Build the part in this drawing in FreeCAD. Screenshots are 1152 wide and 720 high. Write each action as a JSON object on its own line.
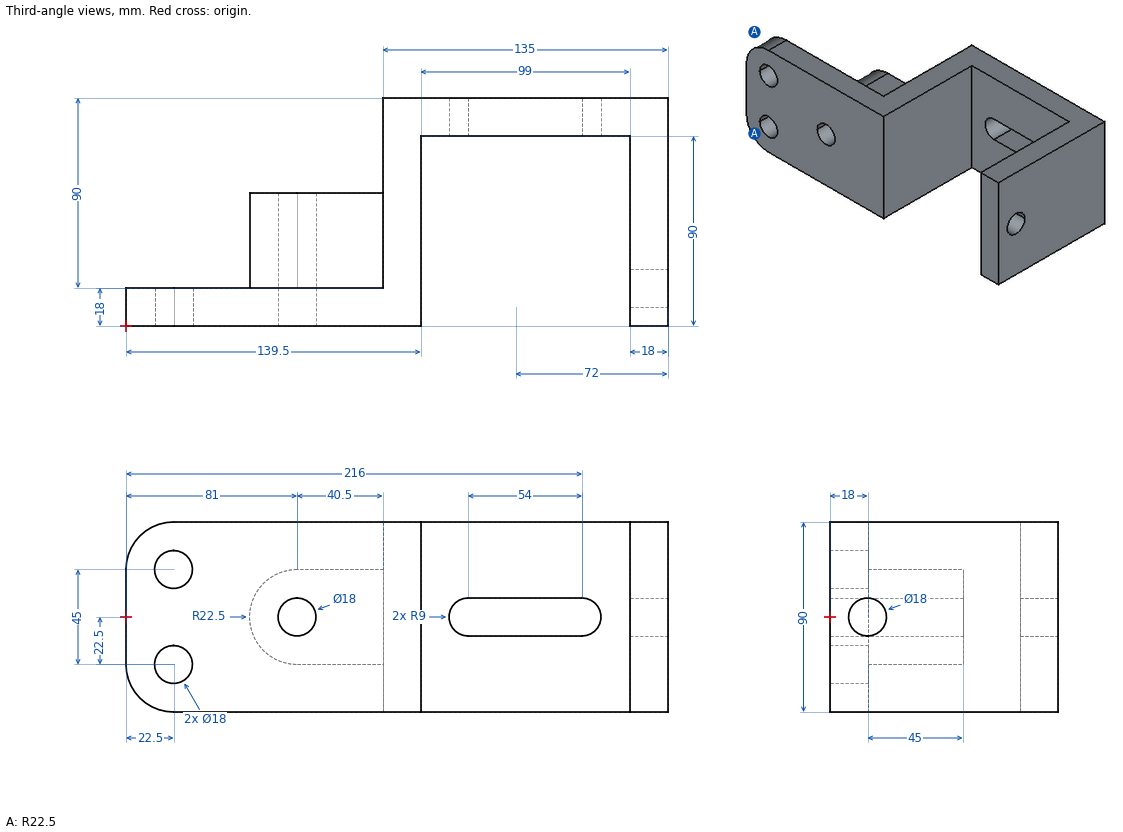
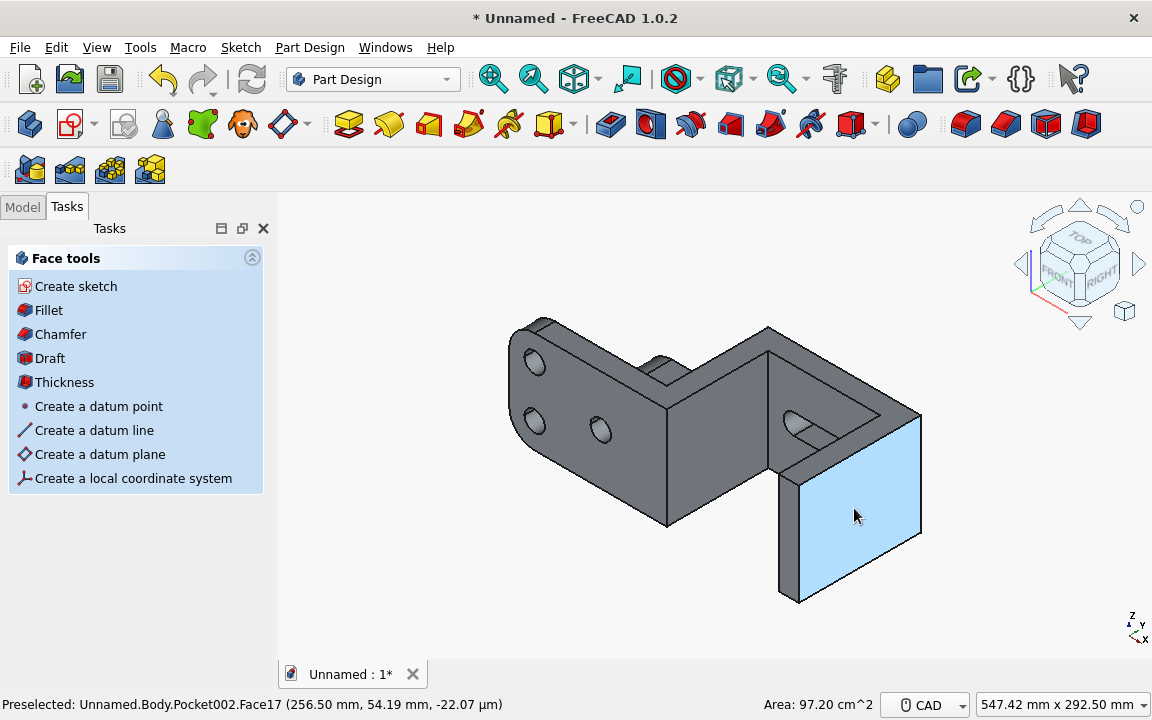
{"action": "left_click", "coordinate": [70, 124]}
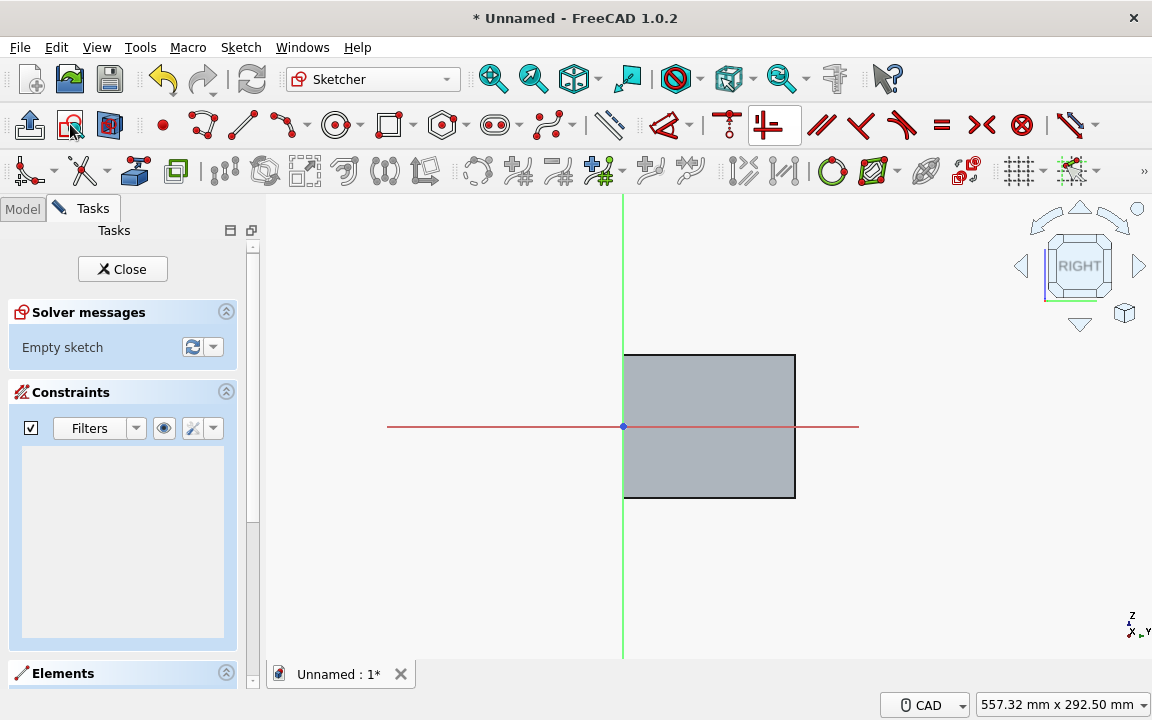
{"action": "scroll", "coordinate": [645, 427], "scroll_direction": "up", "scroll_amount": 12}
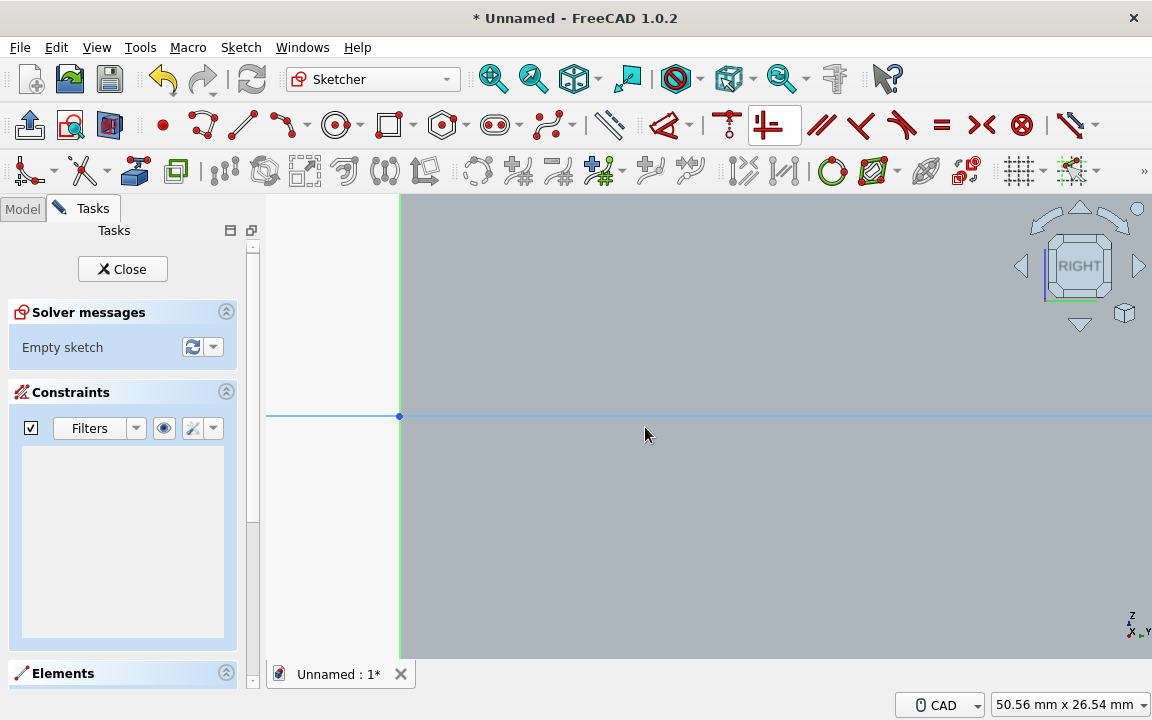
{"action": "left_click", "coordinate": [336, 126]}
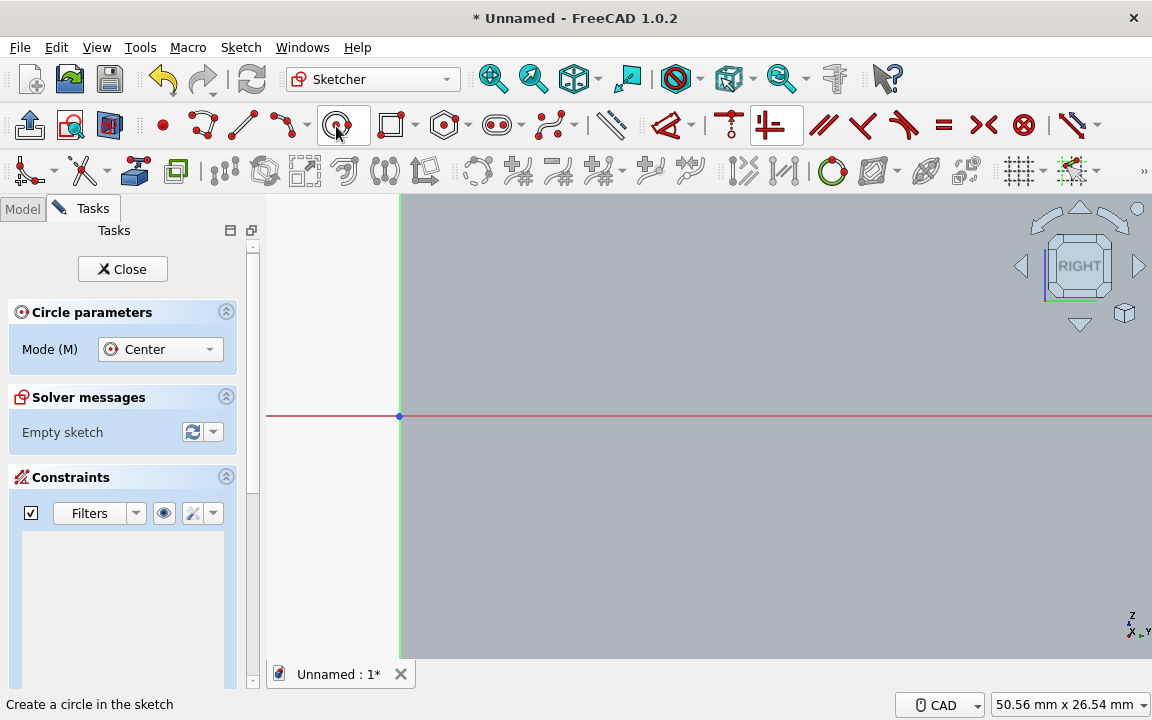
{"action": "left_click", "coordinate": [715, 416]}
{"action": "mouse_move", "coordinate": [827, 305]}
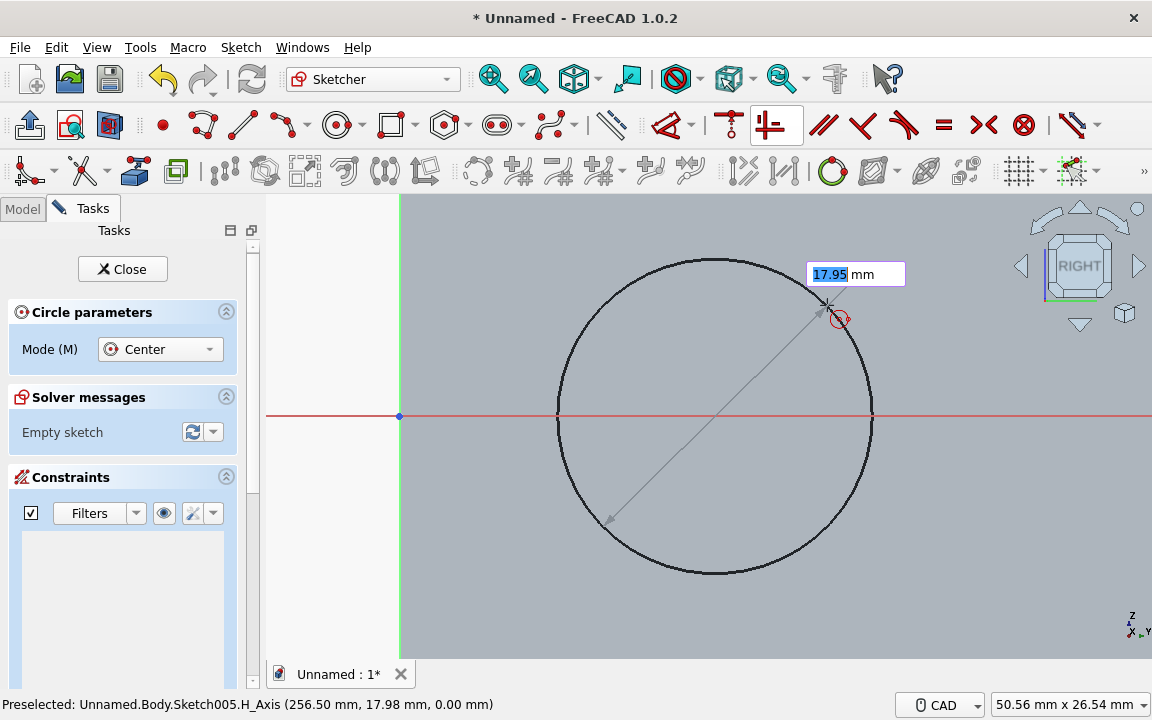
{"action": "type", "text": "18"}
{"action": "key", "text": "Return"}
{"action": "key", "text": "Escape"}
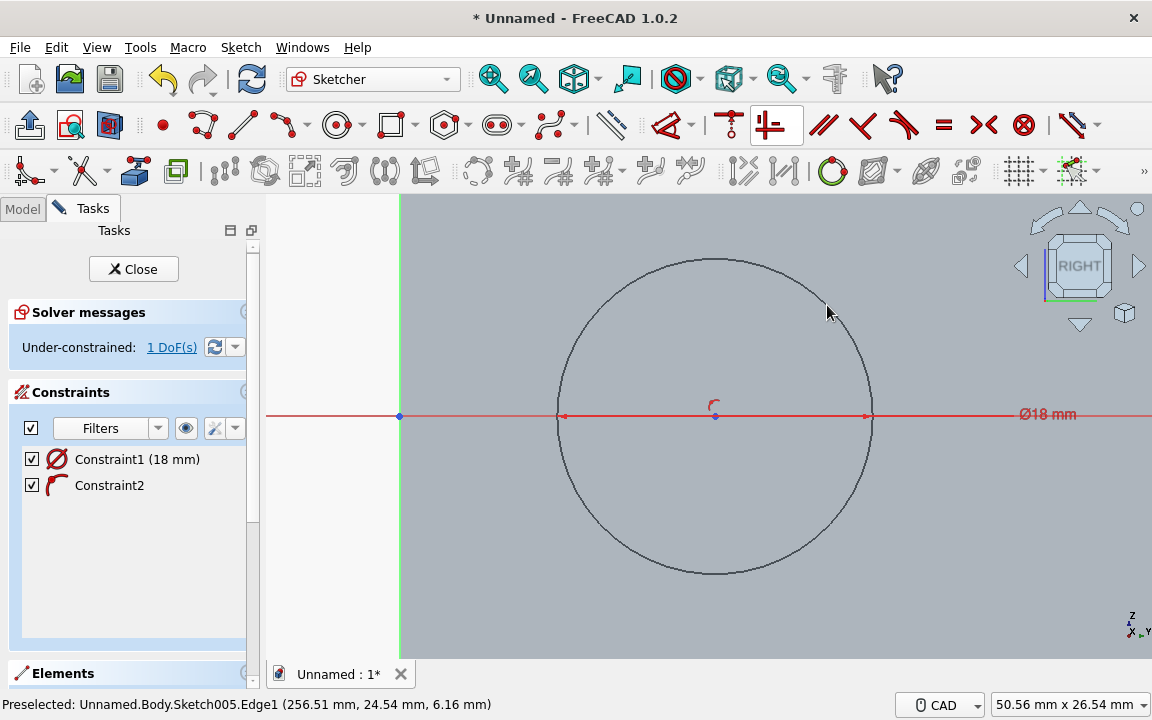
{"action": "left_click", "coordinate": [666, 126]}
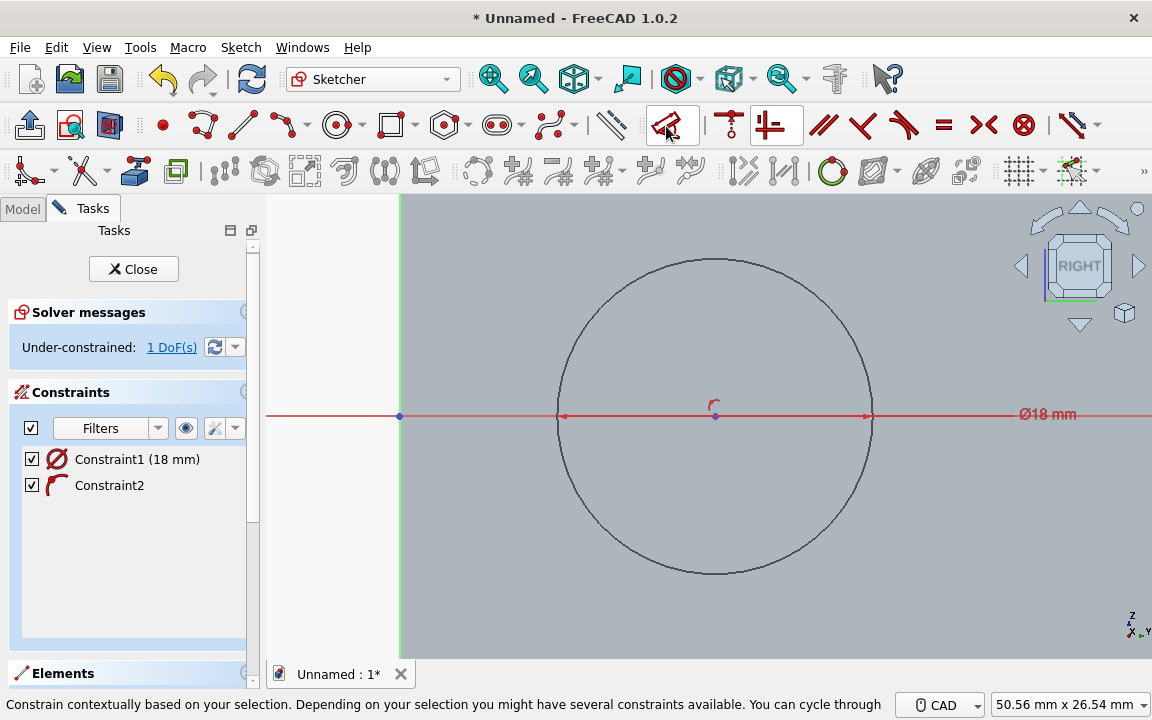
{"action": "left_click", "coordinate": [715, 416]}
{"action": "left_click", "coordinate": [485, 450]}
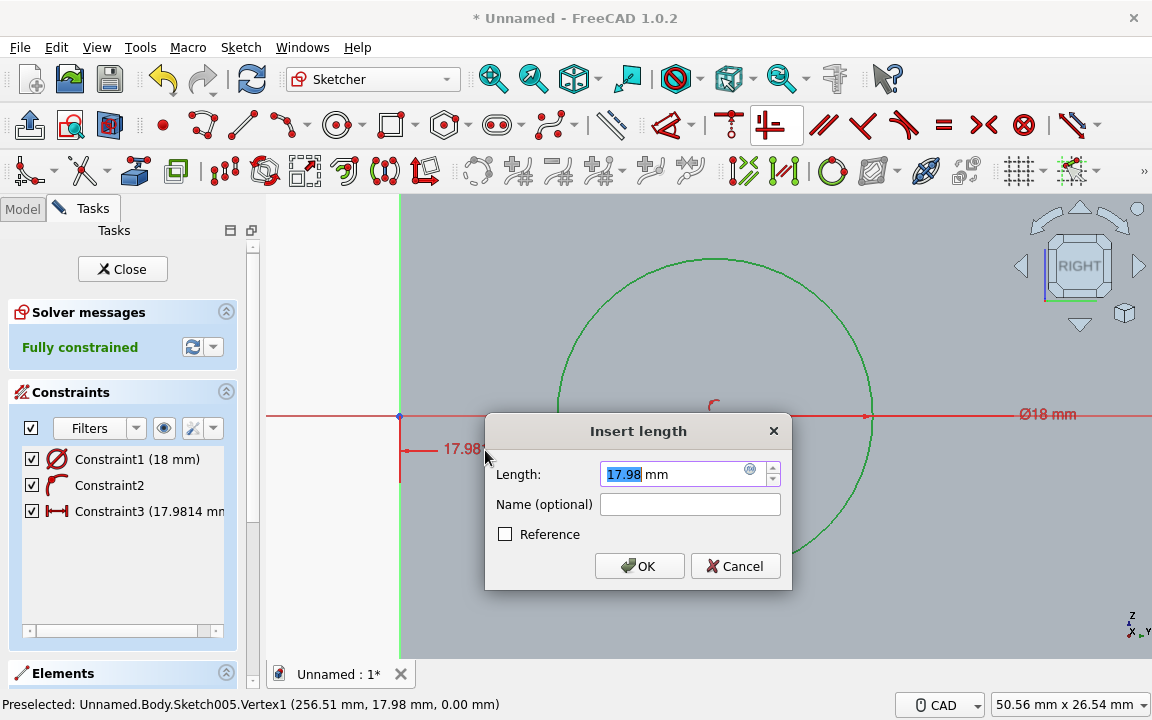
{"action": "type", "text": "18"}
{"action": "key", "text": "Return"}
{"action": "key", "text": "Escape"}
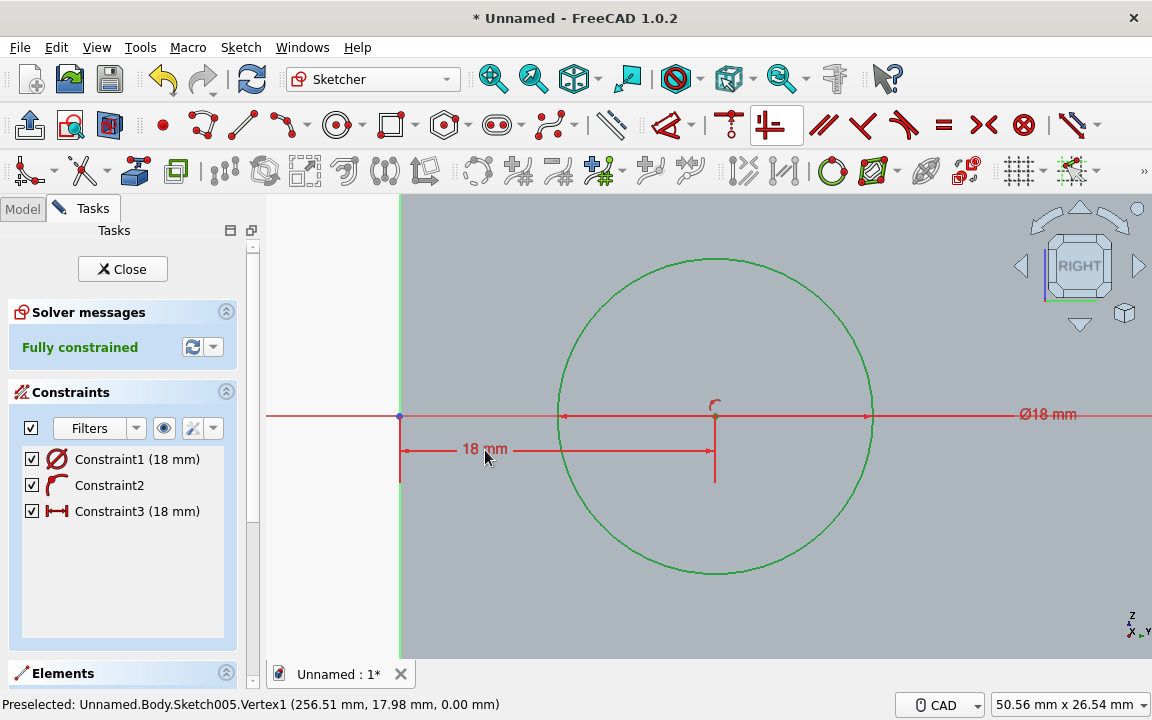
{"action": "left_click", "coordinate": [123, 269]}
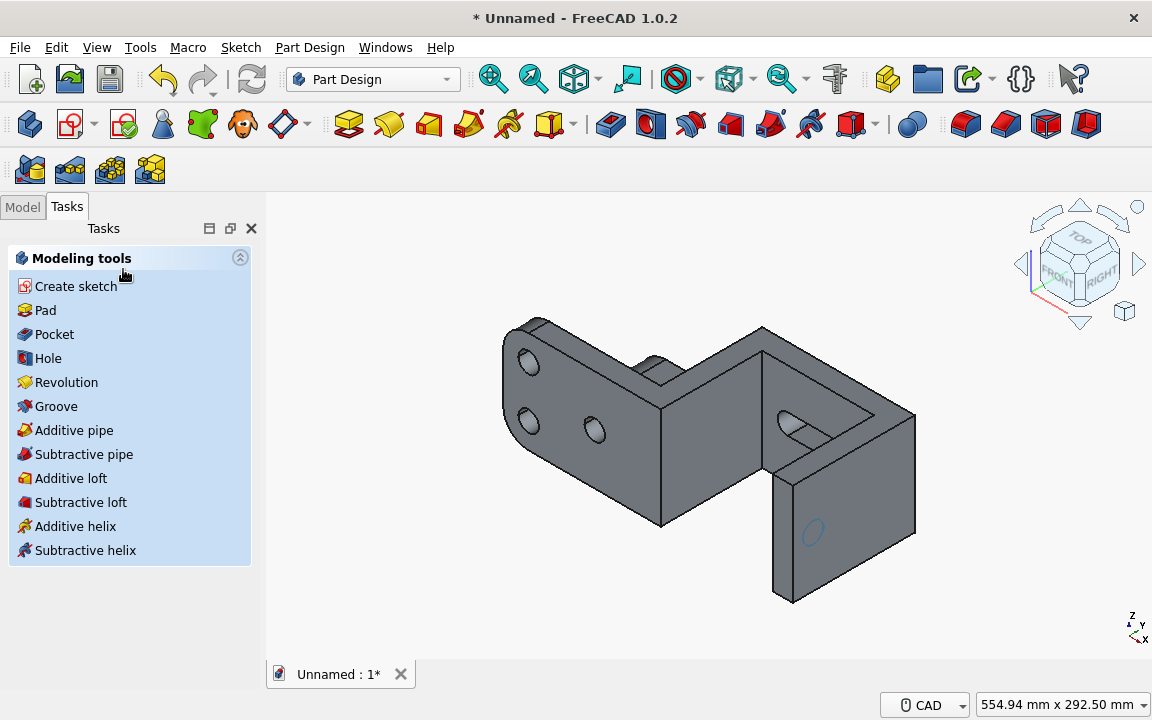
{"action": "left_click", "coordinate": [612, 124]}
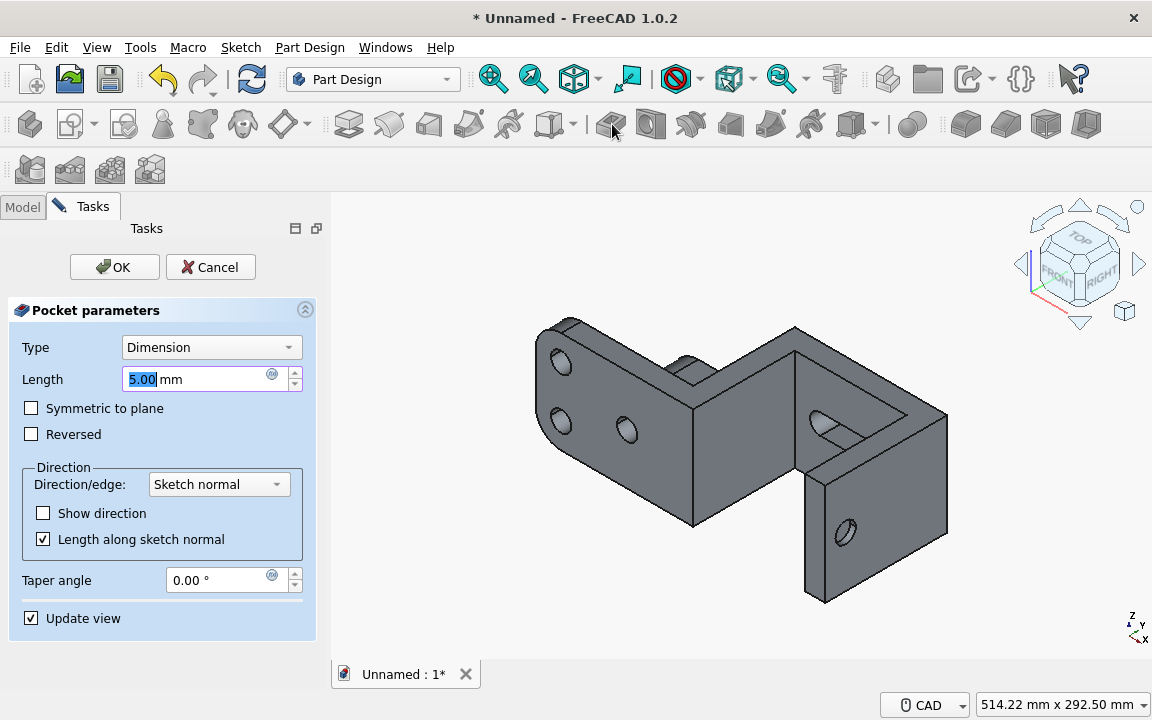
{"action": "type", "text": "72"}
{"action": "key", "text": "Tab"}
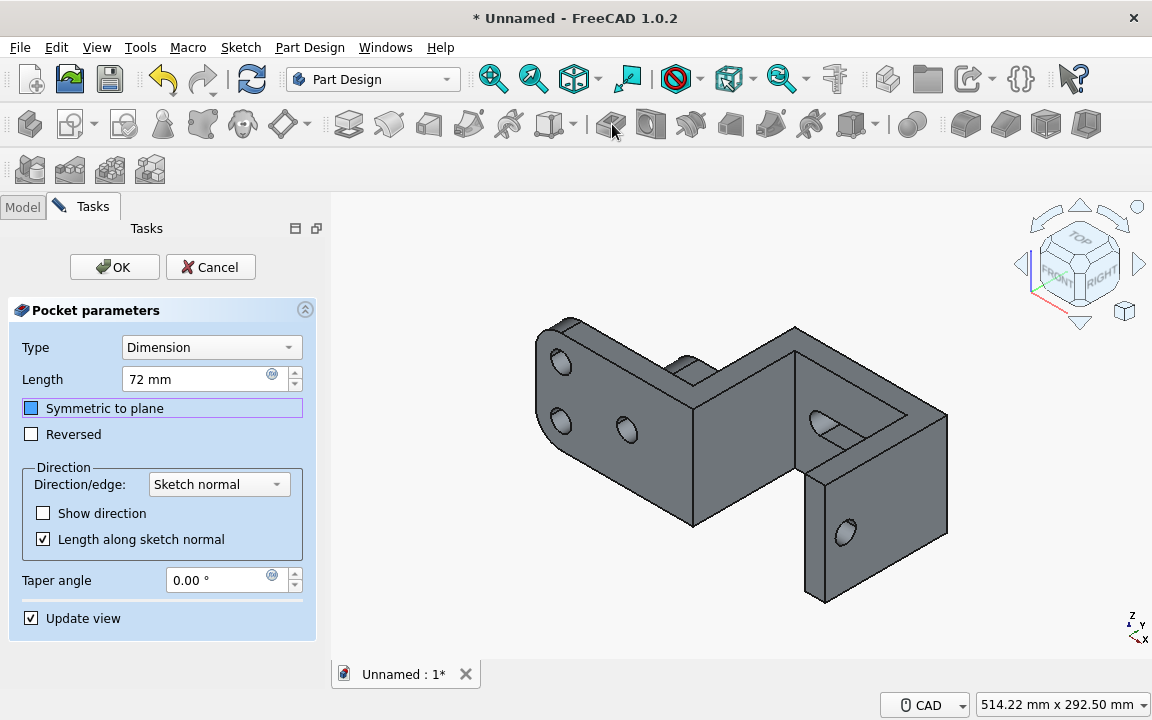
{"action": "left_click", "coordinate": [115, 267]}